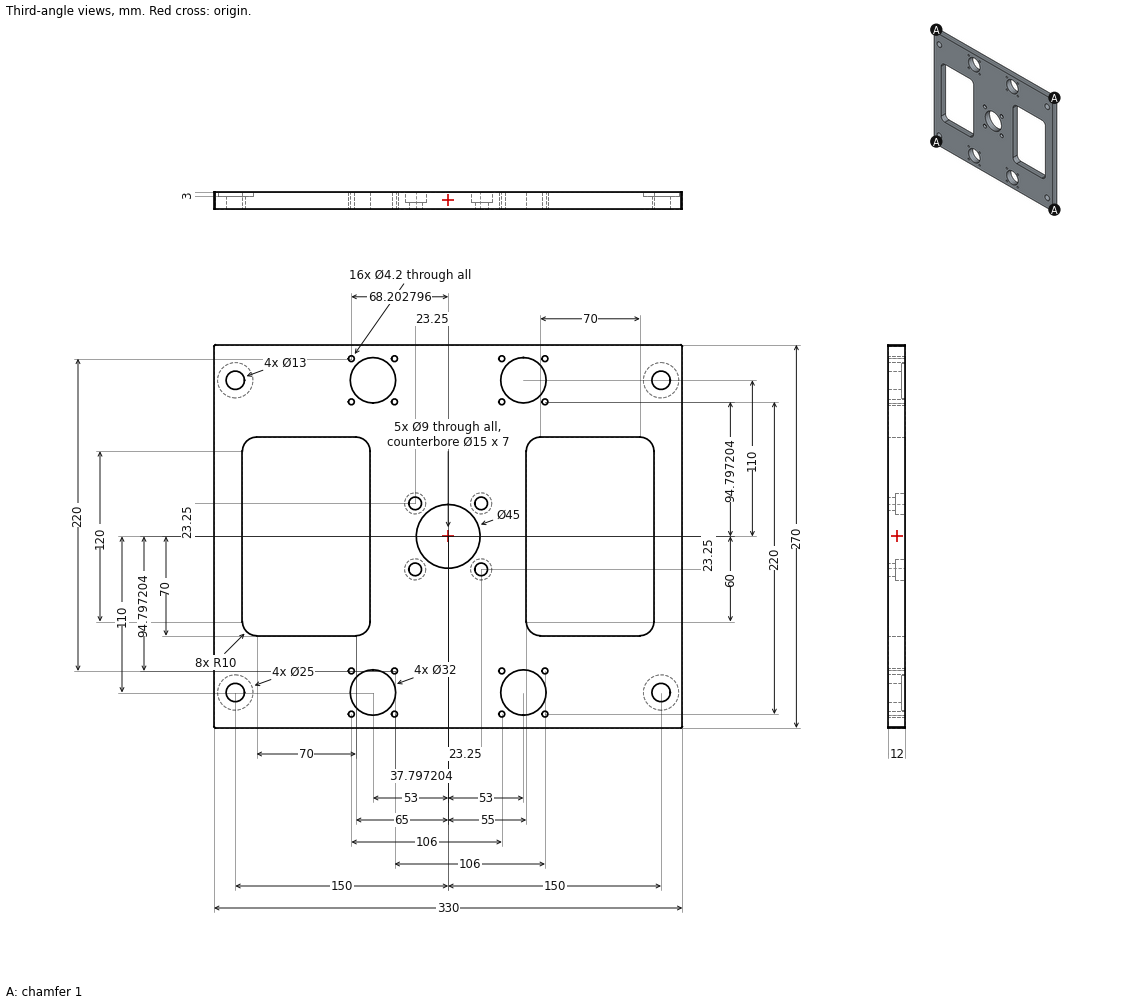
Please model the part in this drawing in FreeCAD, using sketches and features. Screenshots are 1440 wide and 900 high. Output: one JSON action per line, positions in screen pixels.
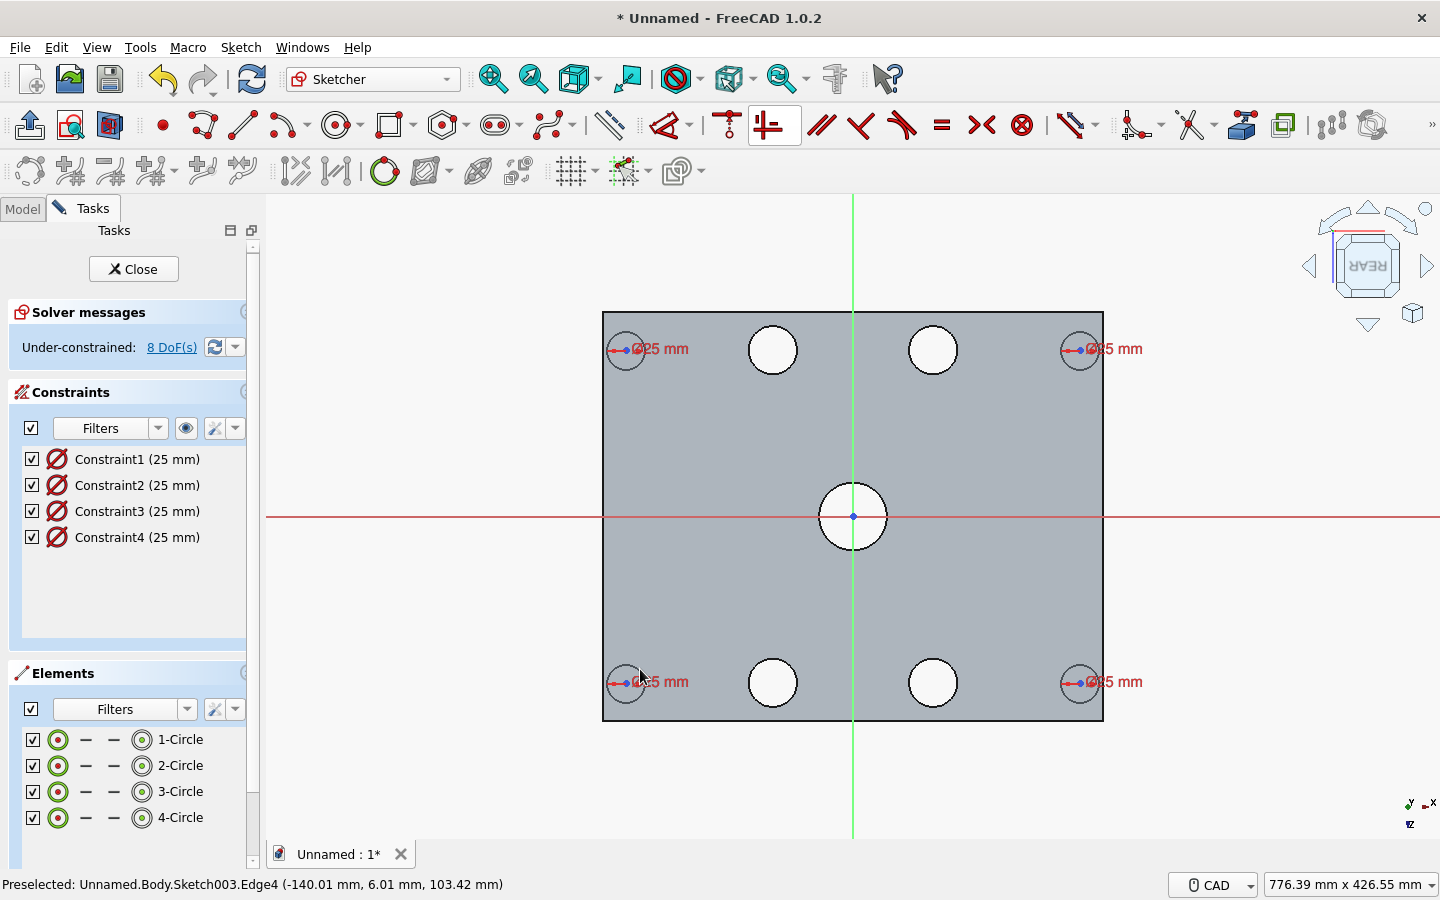
{"action": "left_click", "coordinate": [626, 351]}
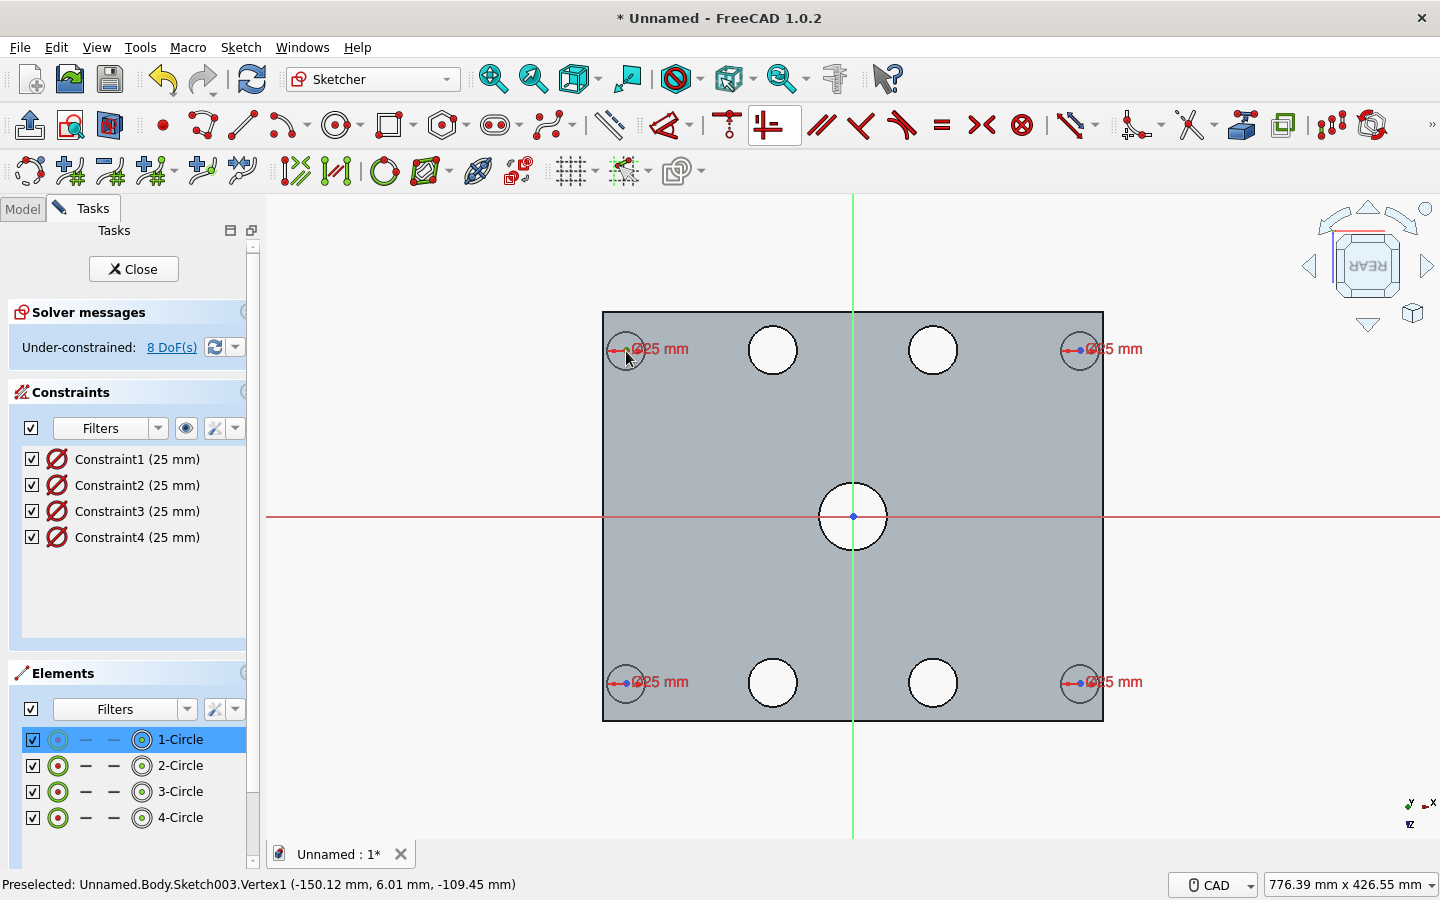
{"action": "left_click", "coordinate": [1080, 351]}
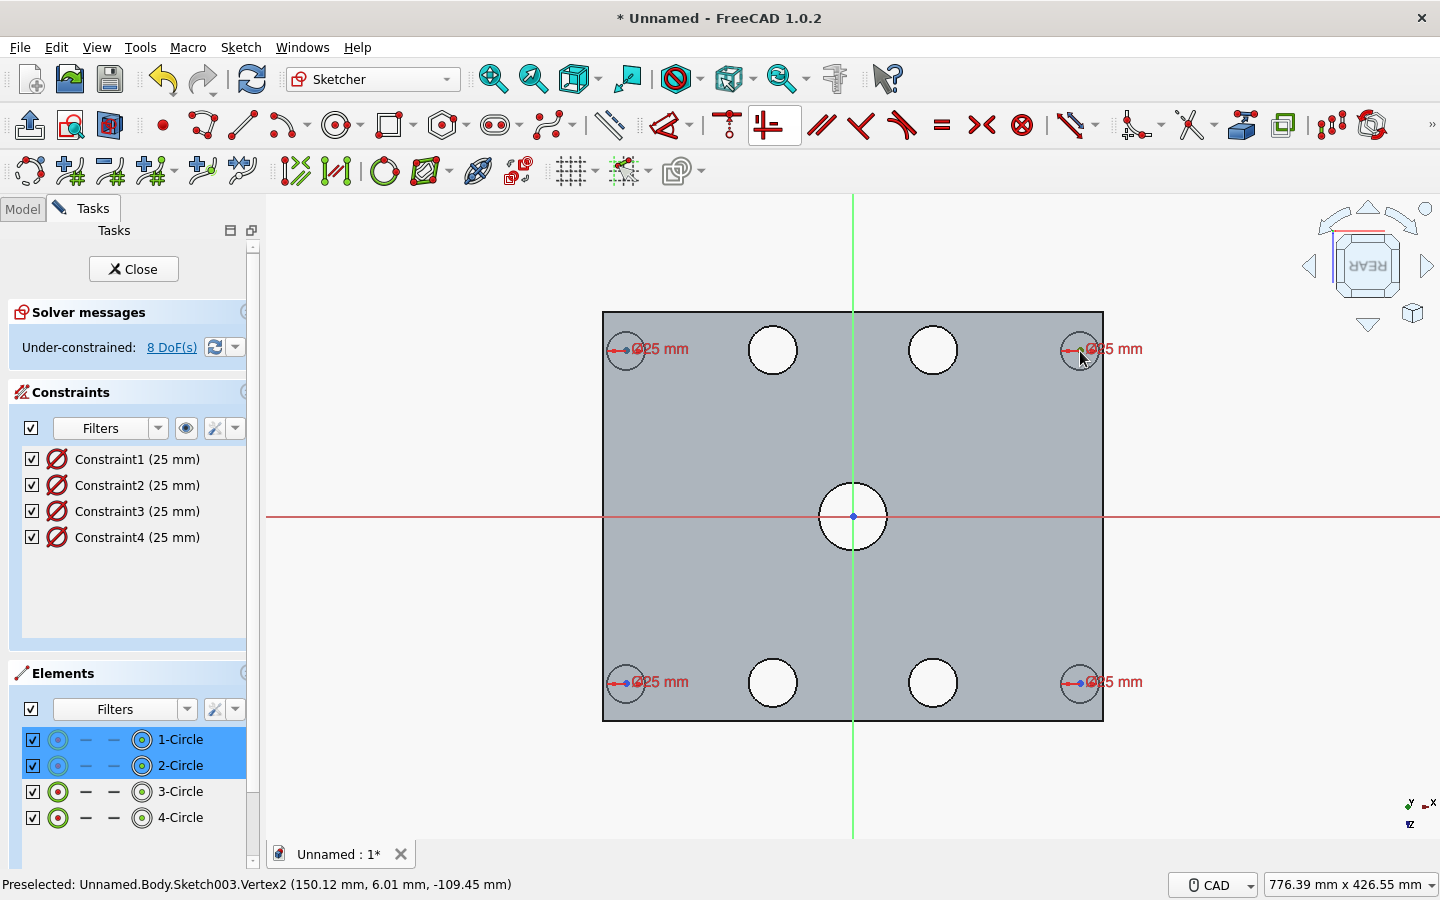
{"action": "key", "text": "h"}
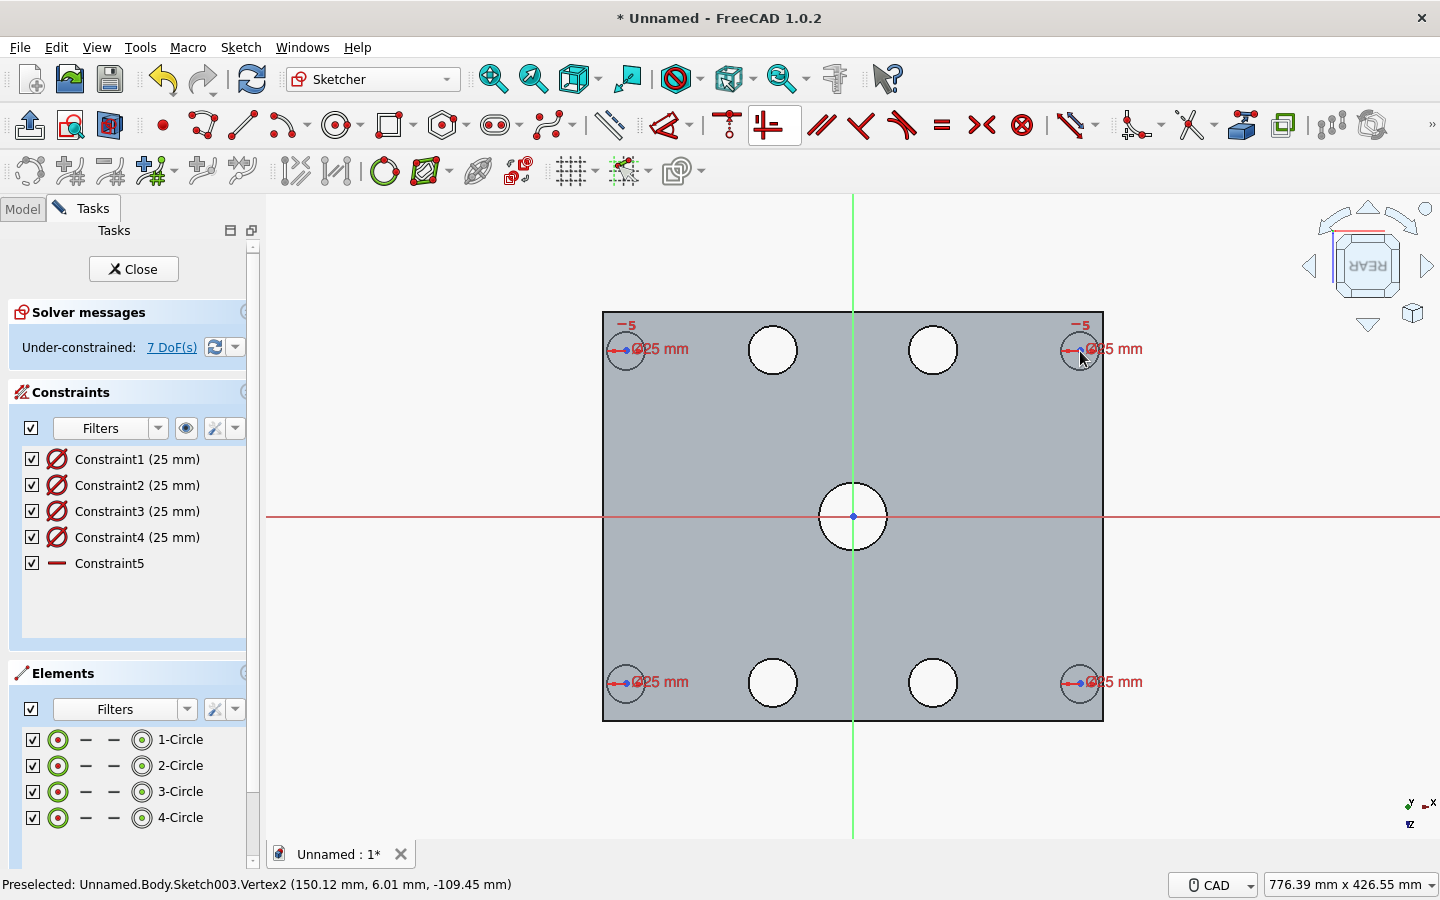
{"action": "left_click", "coordinate": [1080, 351]}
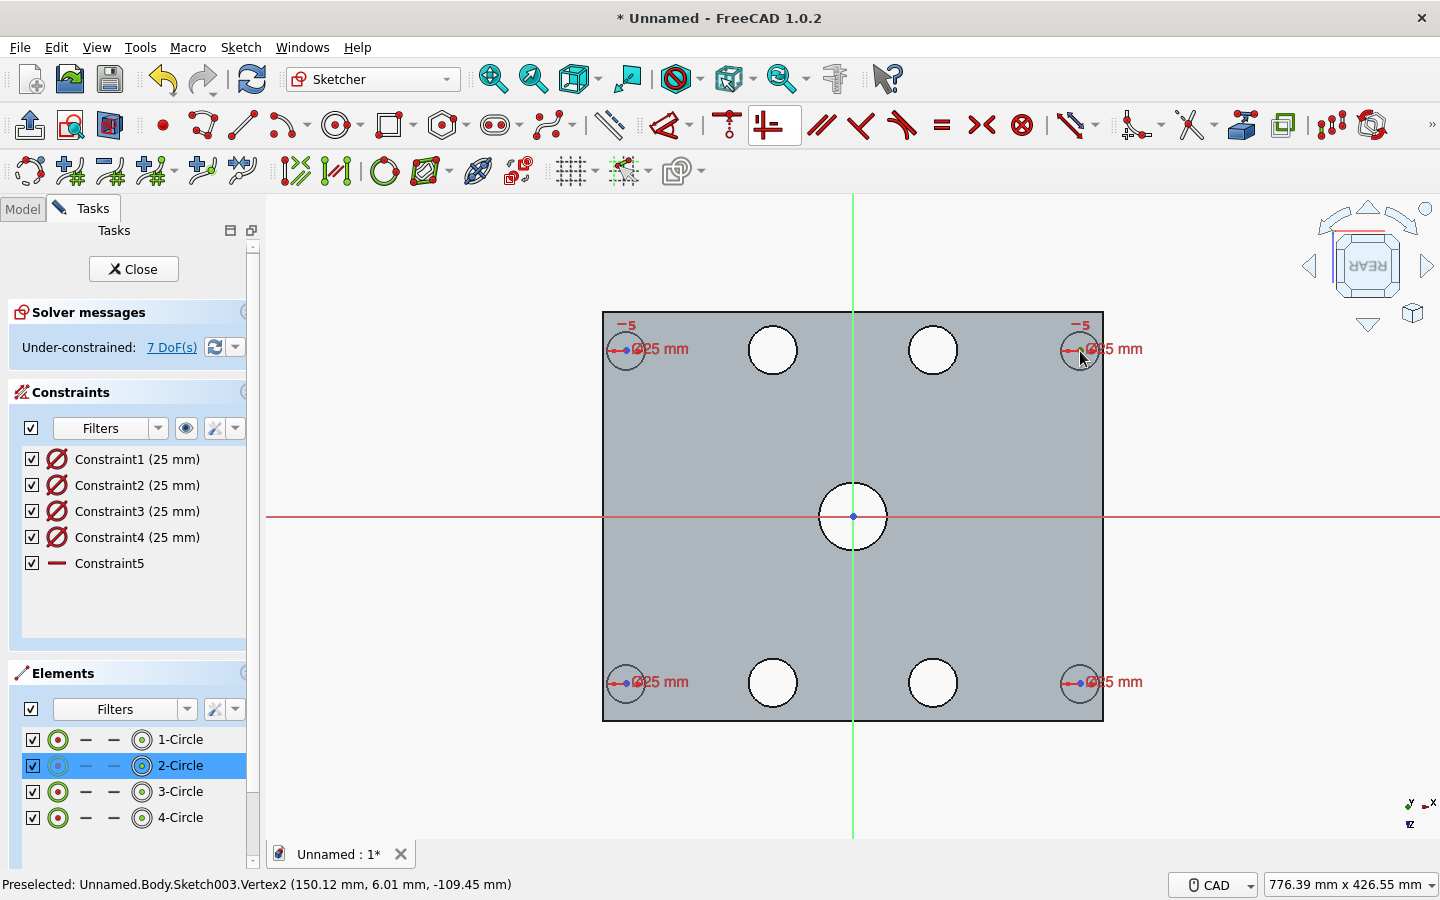
{"action": "left_click", "coordinate": [1080, 684]}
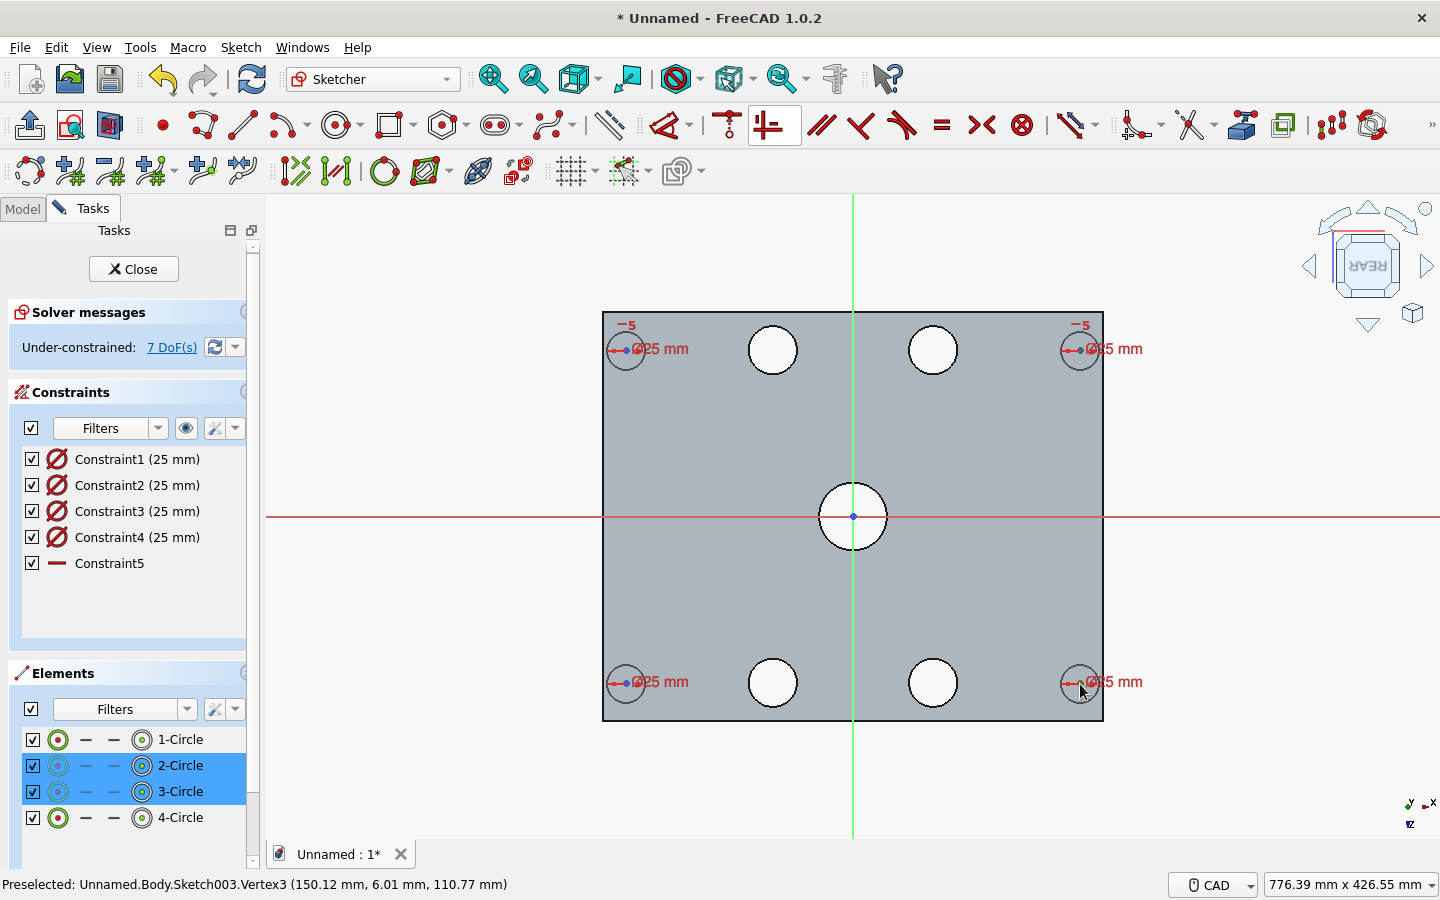
{"action": "left_click", "coordinate": [796, 126]}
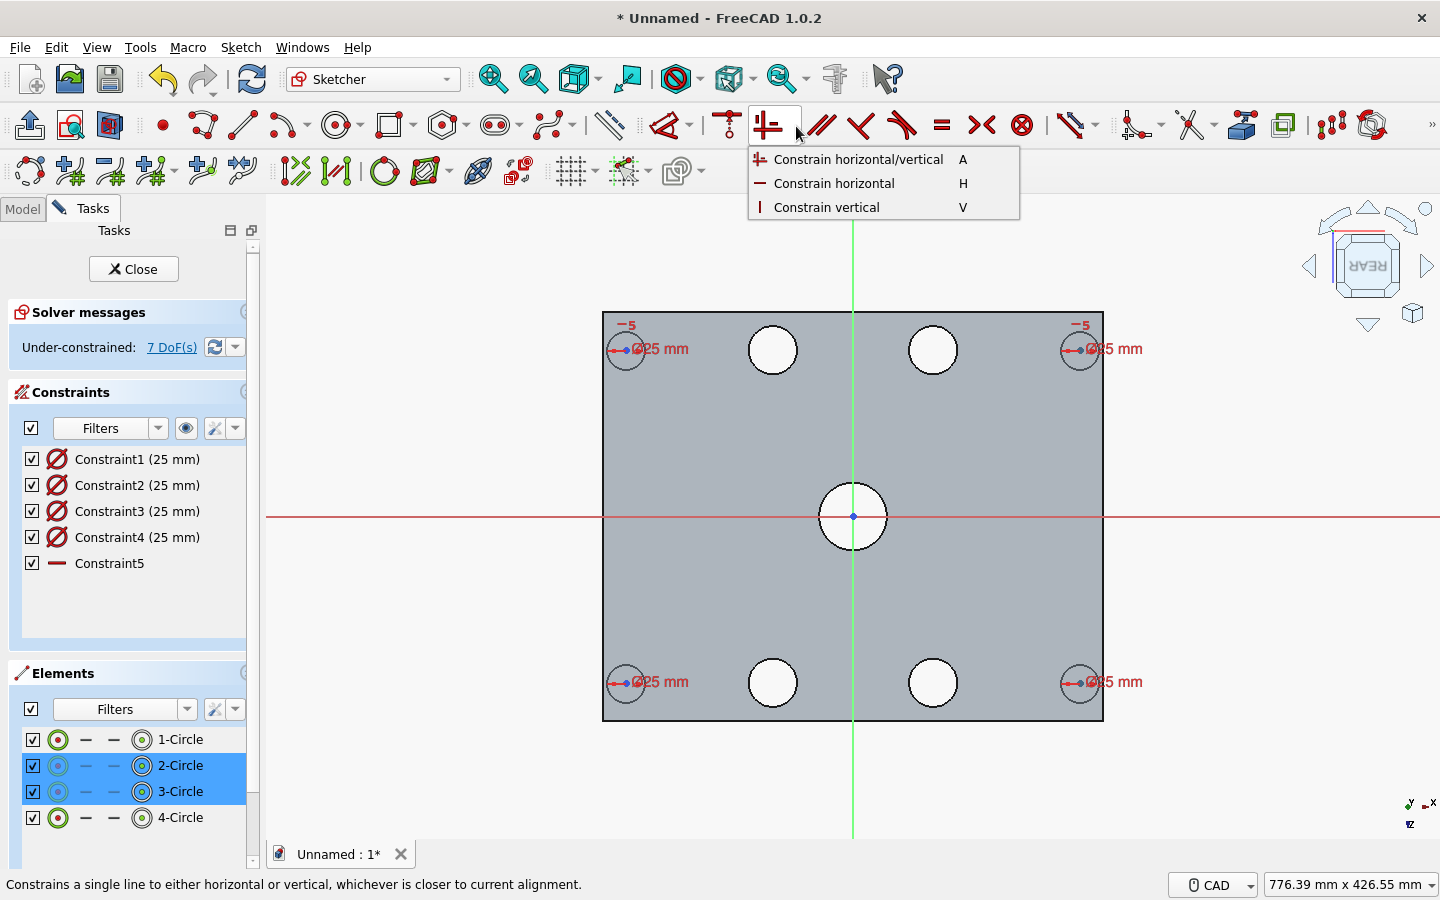
{"action": "left_click", "coordinate": [884, 207]}